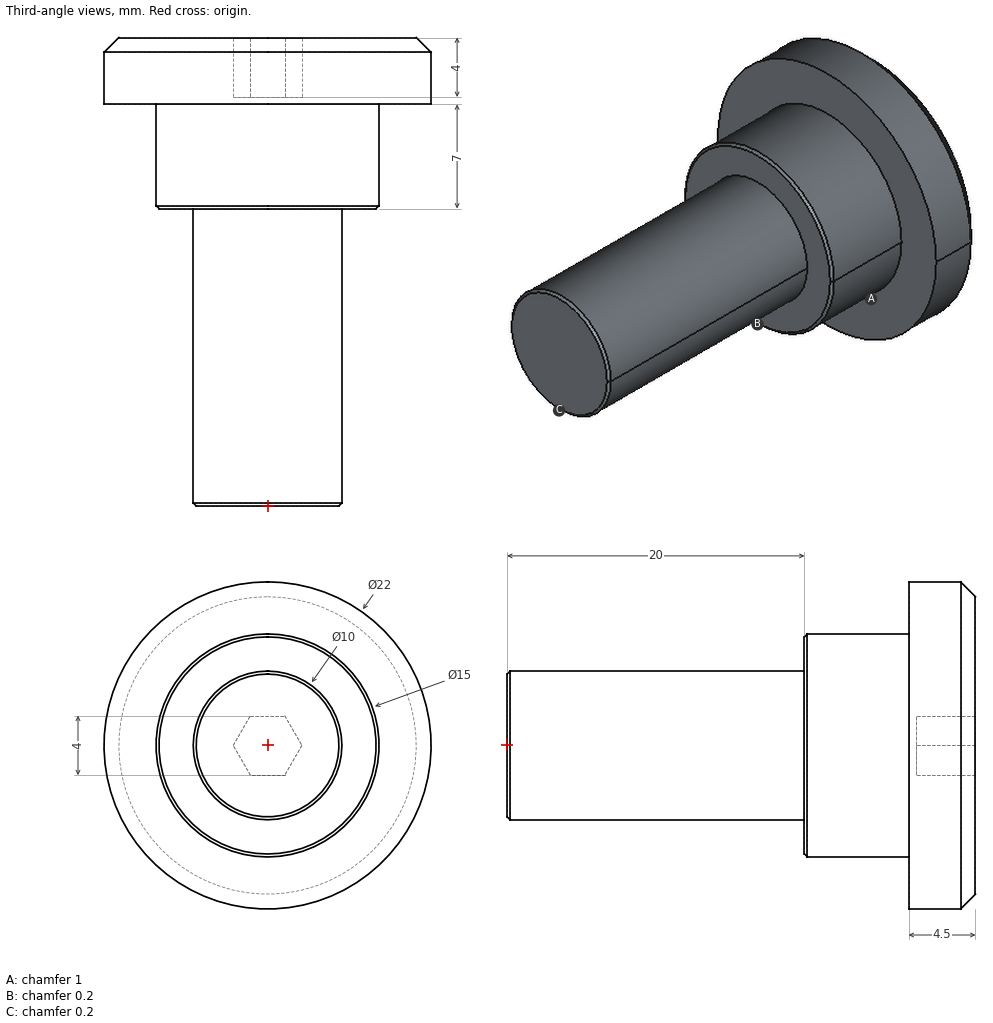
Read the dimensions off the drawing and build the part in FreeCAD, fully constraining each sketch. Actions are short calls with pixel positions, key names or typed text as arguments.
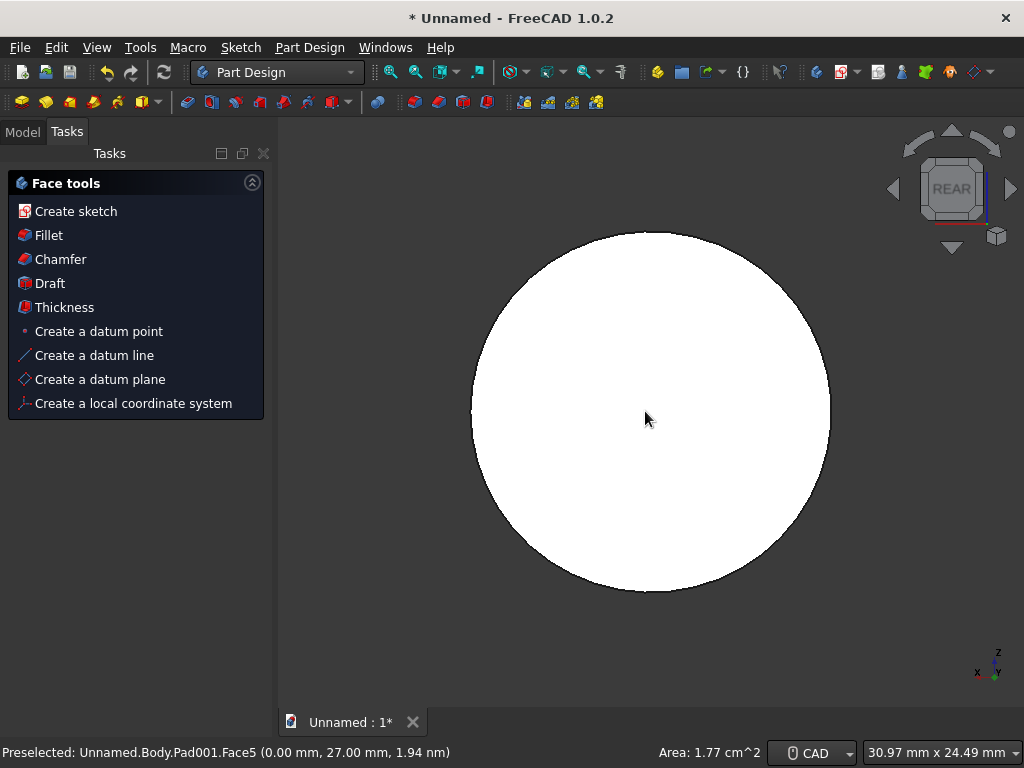
click(842, 72)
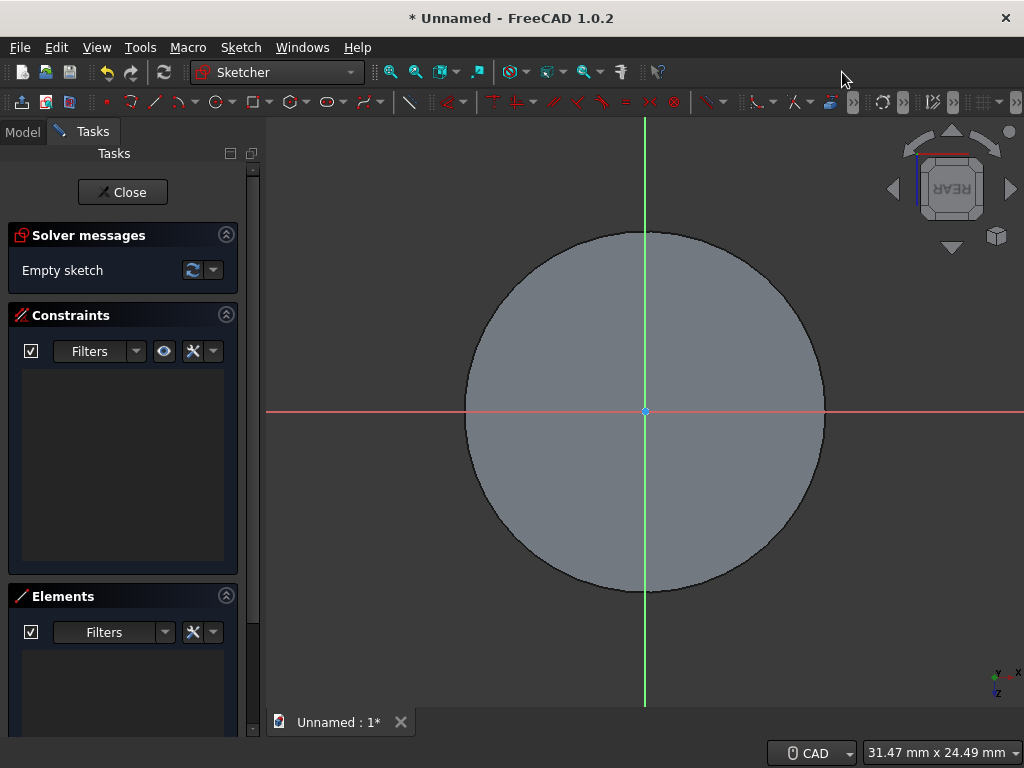
scroll(437, 412, down, 2)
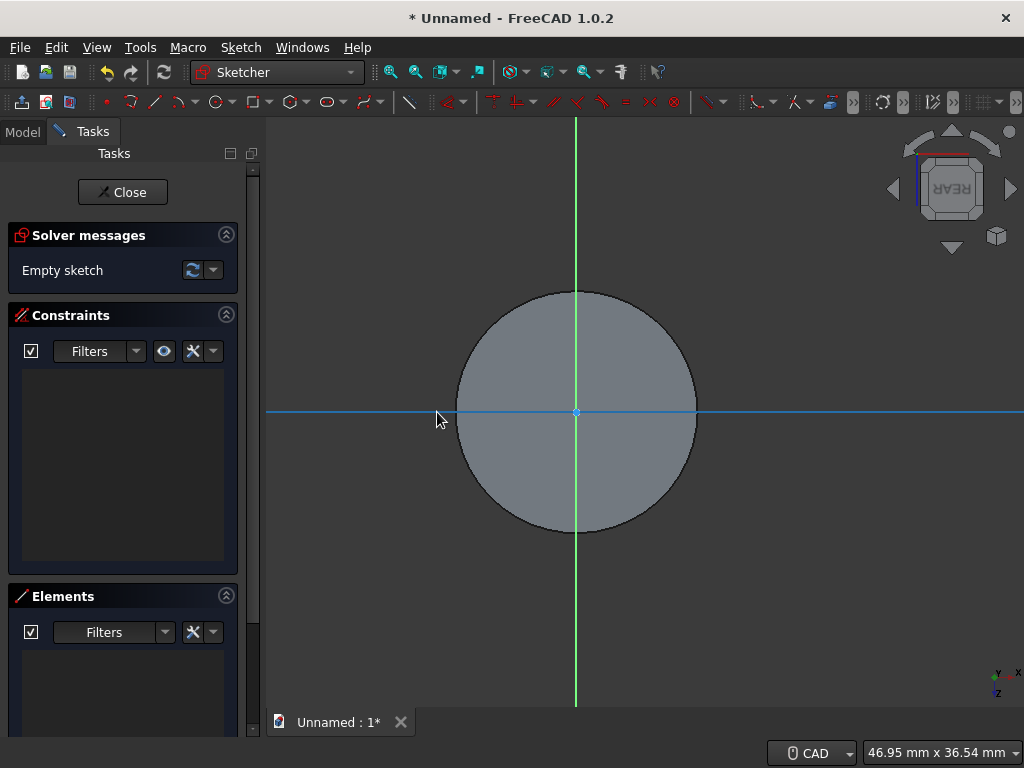
click(216, 102)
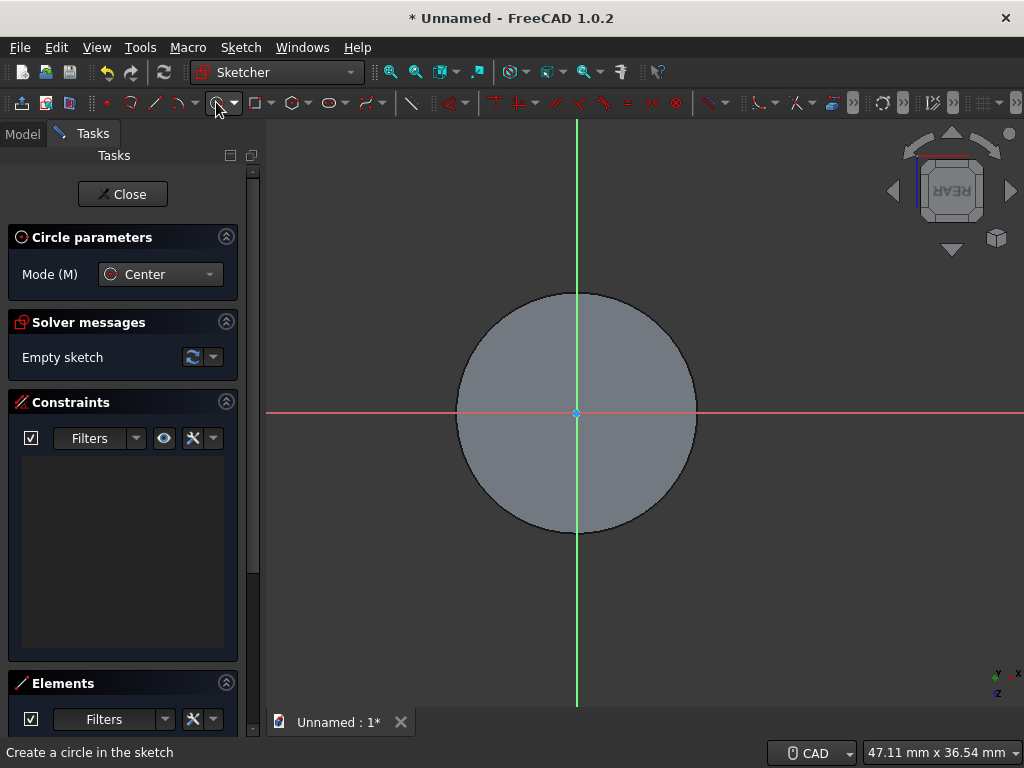
click(577, 413)
move(702, 288)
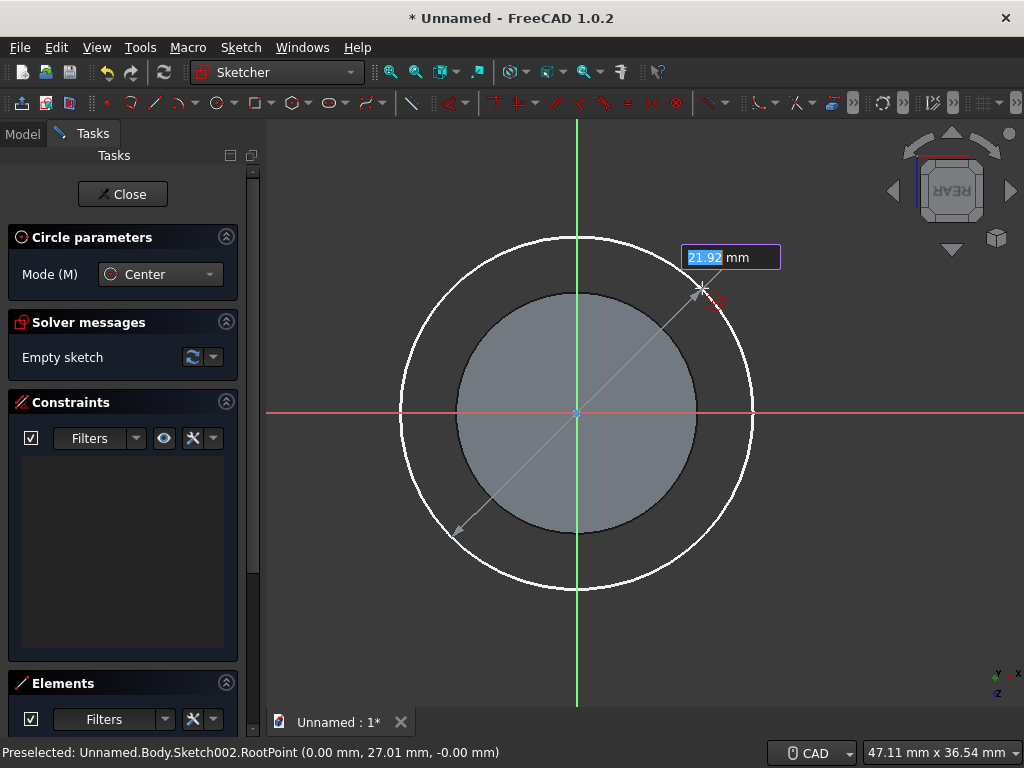
text(22)
key(Return)
key(Escape)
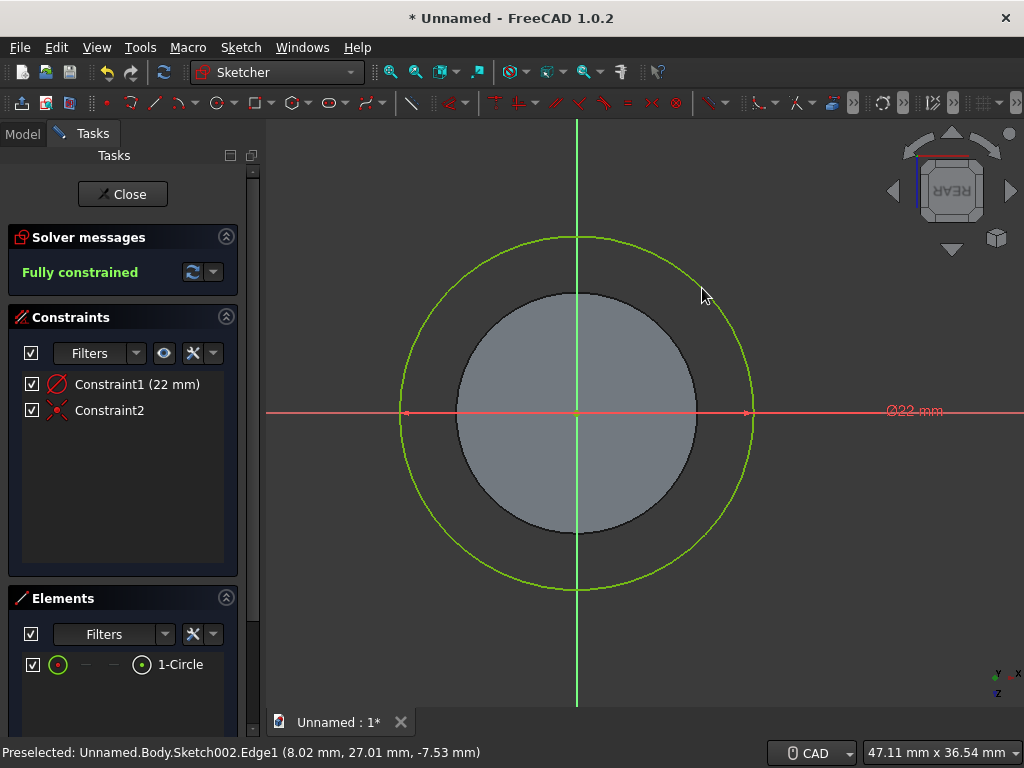
click(123, 194)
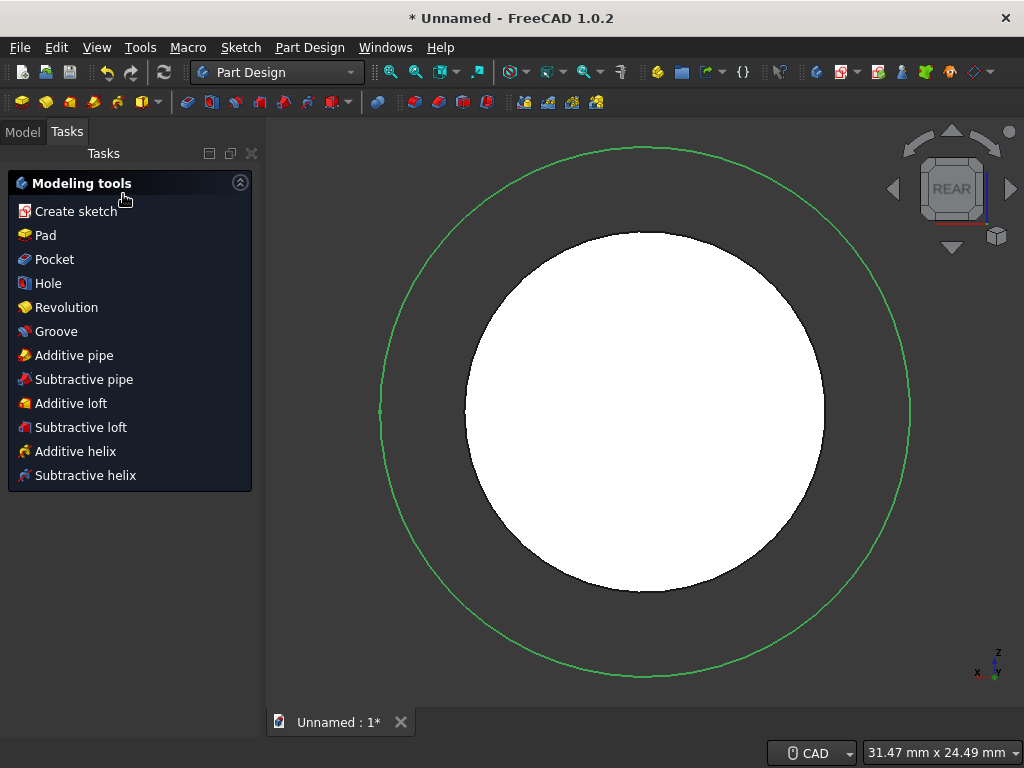
click(22, 102)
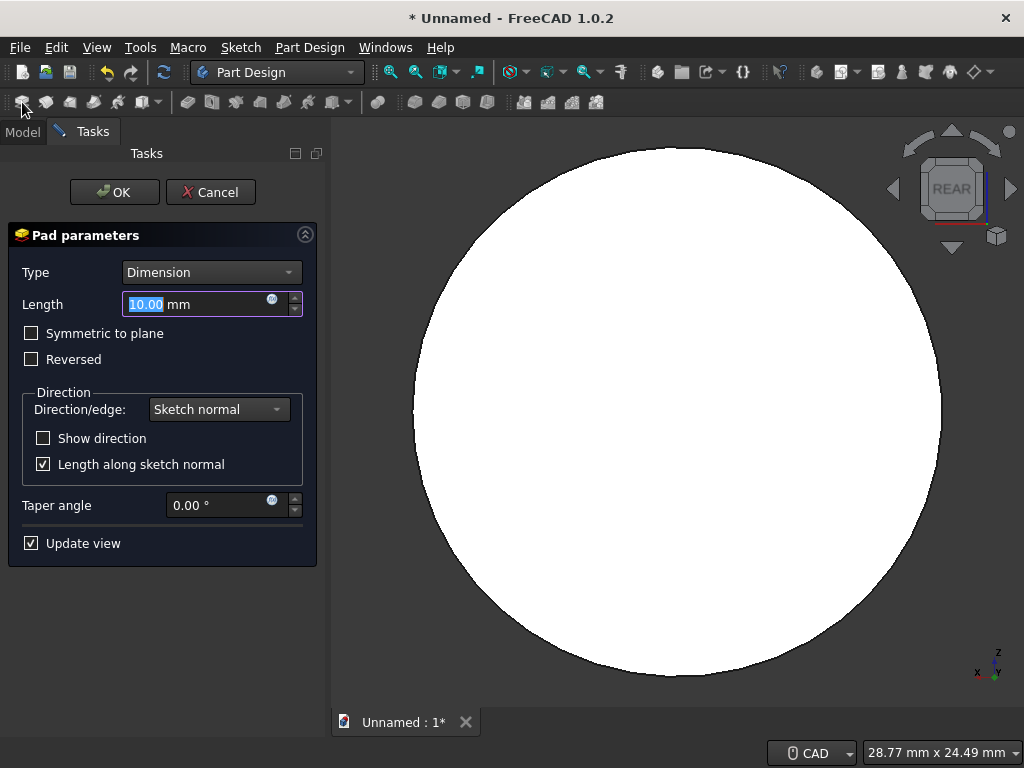
text(4.5)
key(Tab)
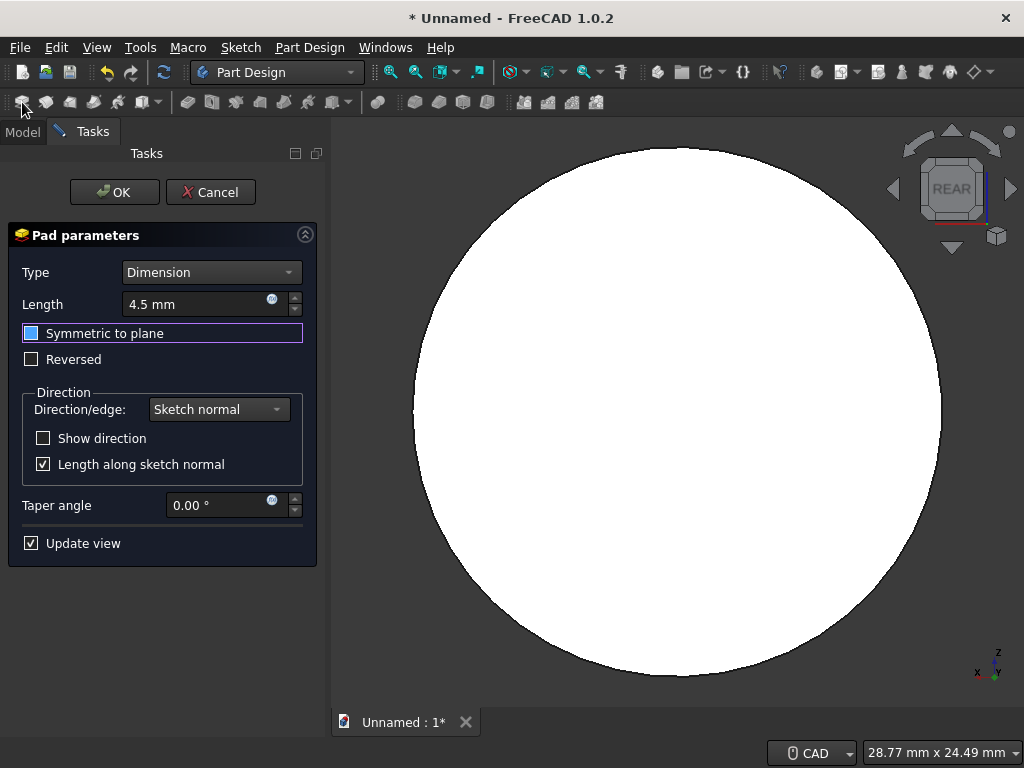
click(115, 192)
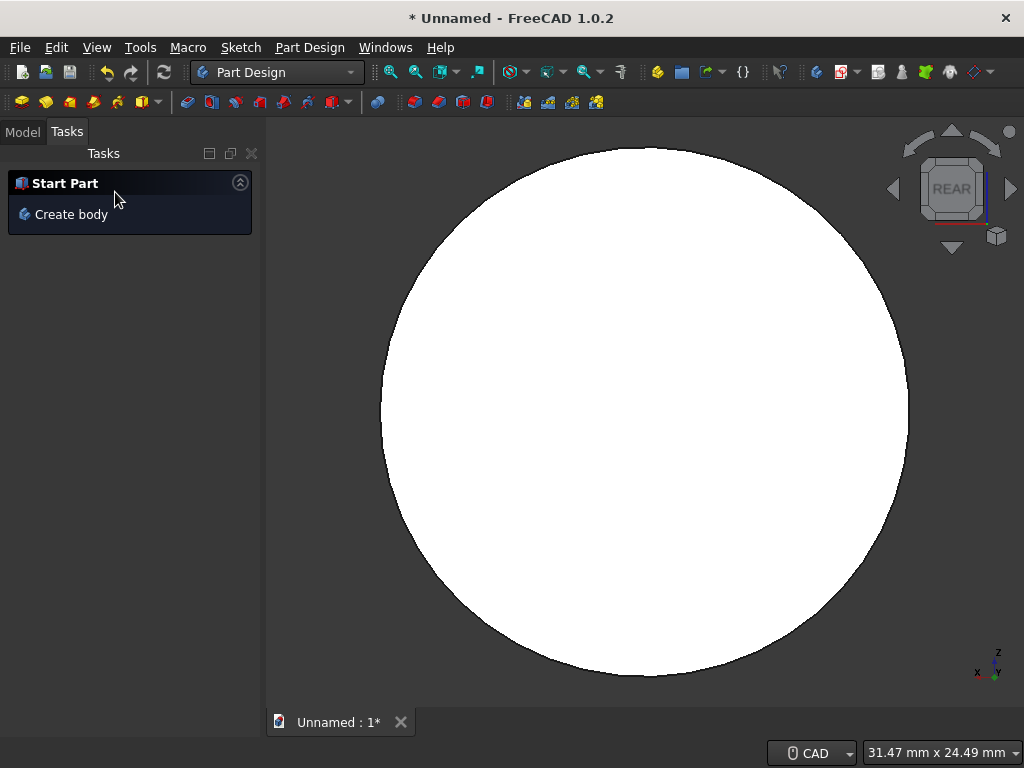
click(910, 411)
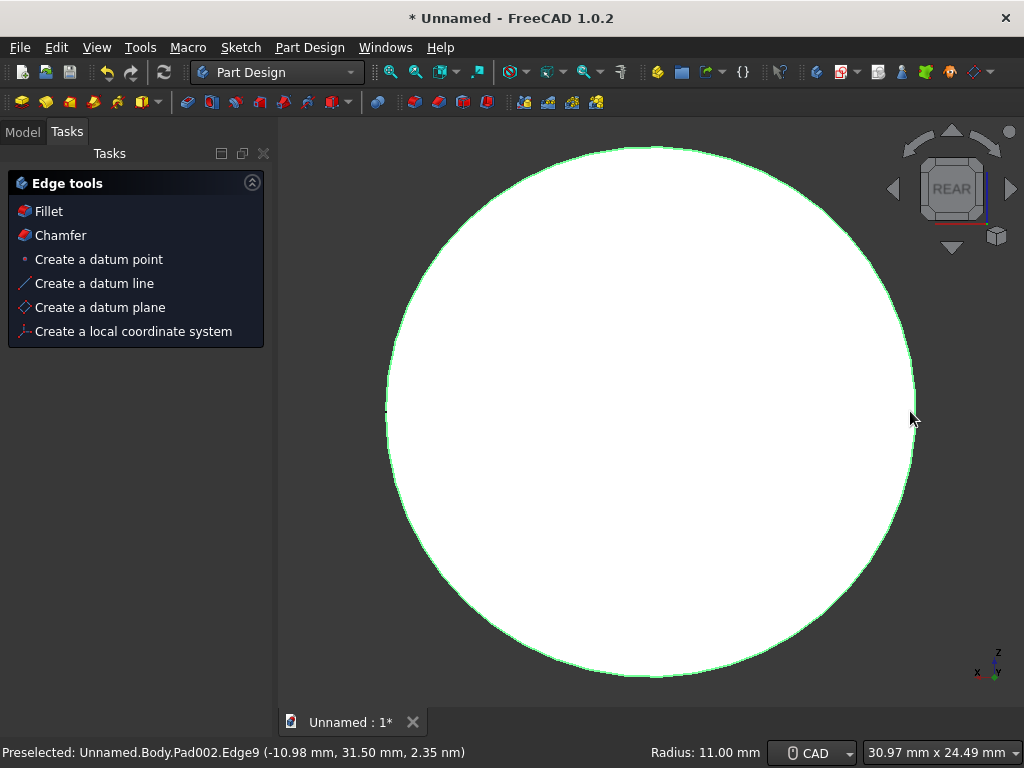
click(440, 102)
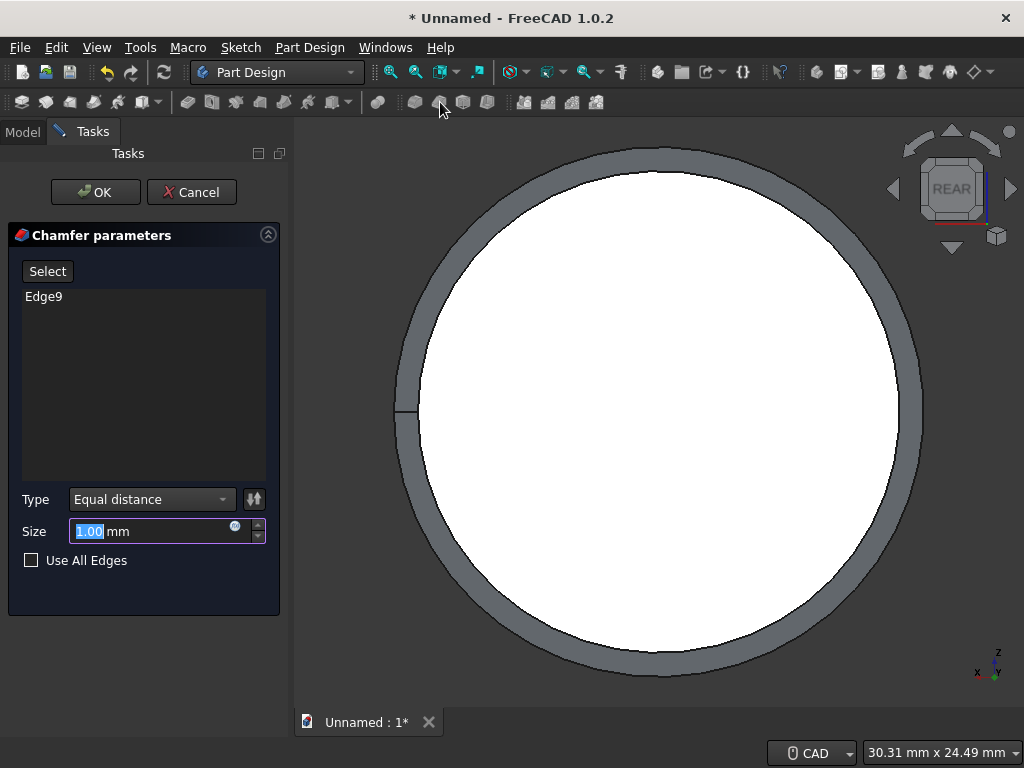
text(1)
key(Tab)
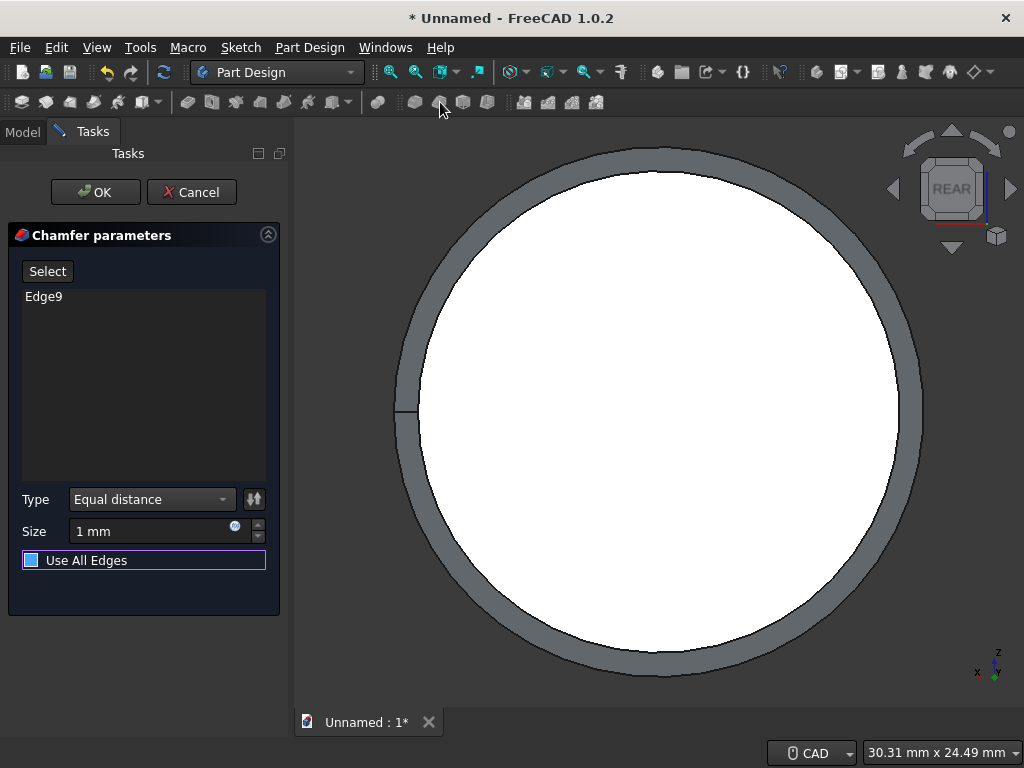
click(96, 192)